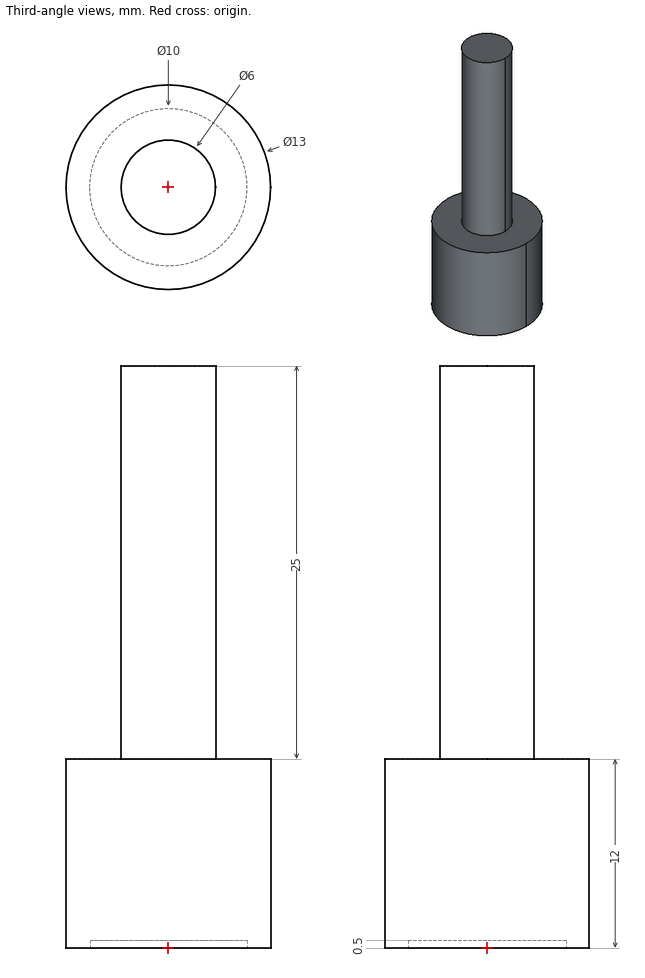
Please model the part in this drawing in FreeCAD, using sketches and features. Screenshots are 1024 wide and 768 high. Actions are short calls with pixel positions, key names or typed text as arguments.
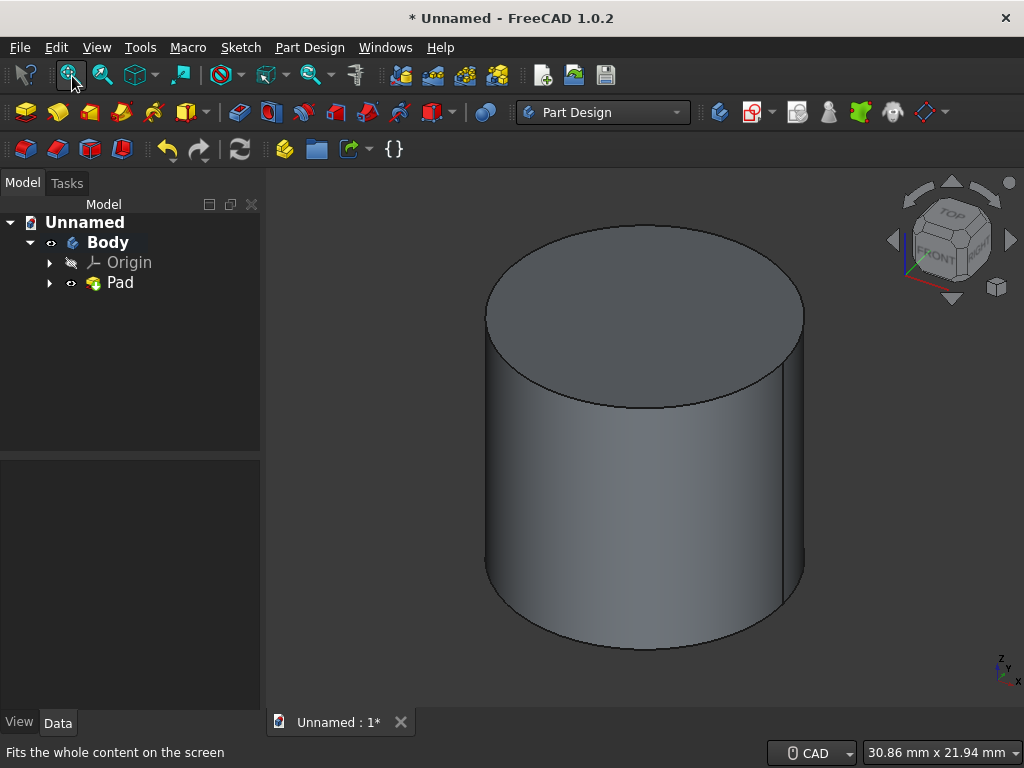
click(645, 316)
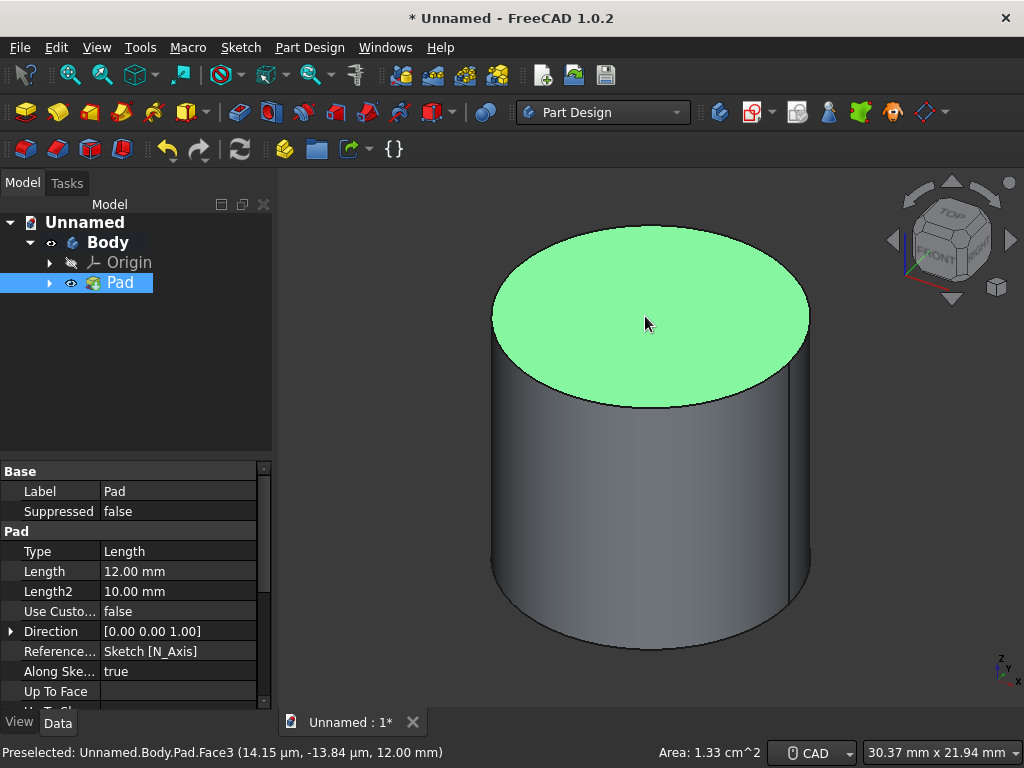
click(752, 112)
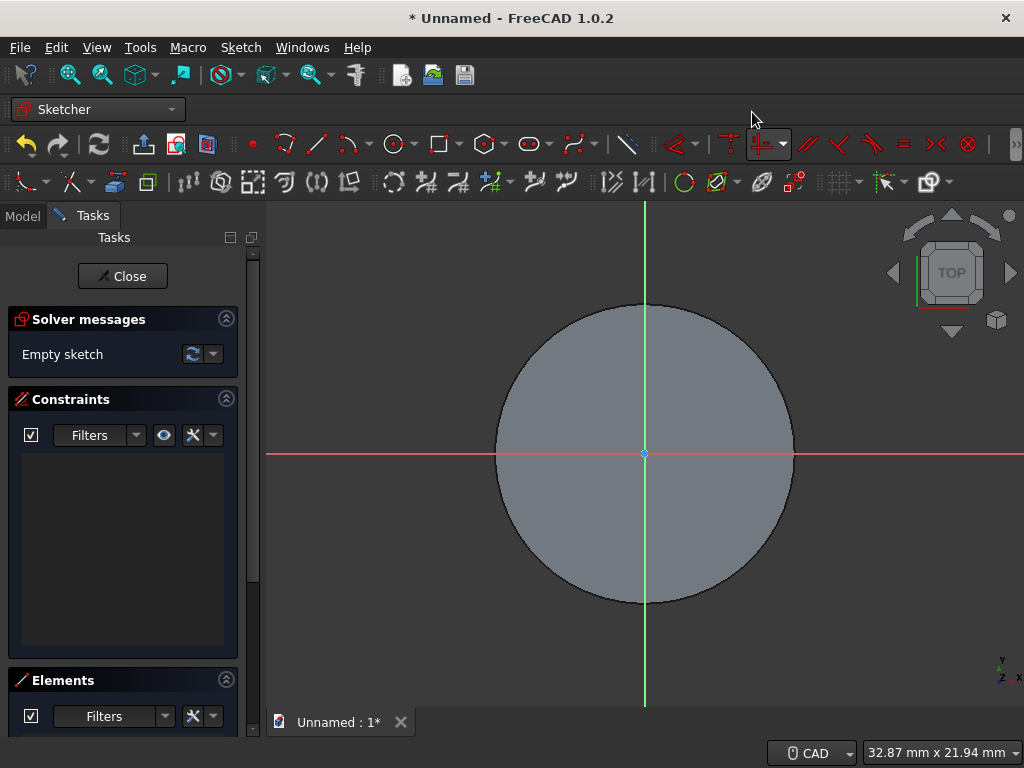
scroll(701, 454, up, 4)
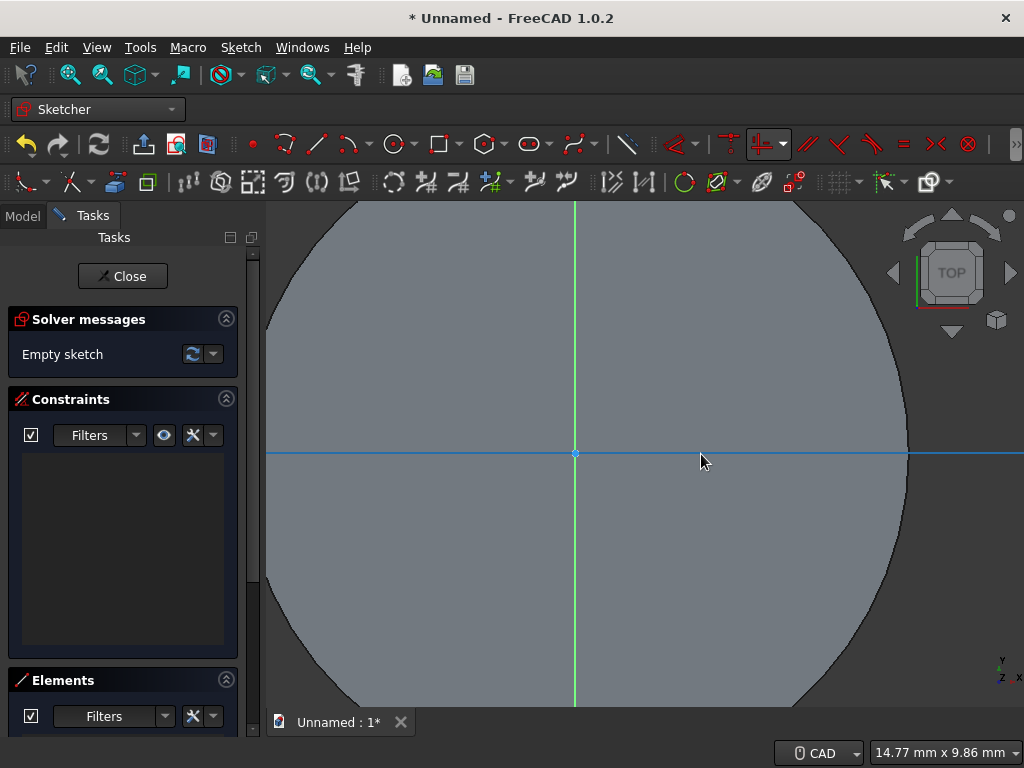
click(394, 144)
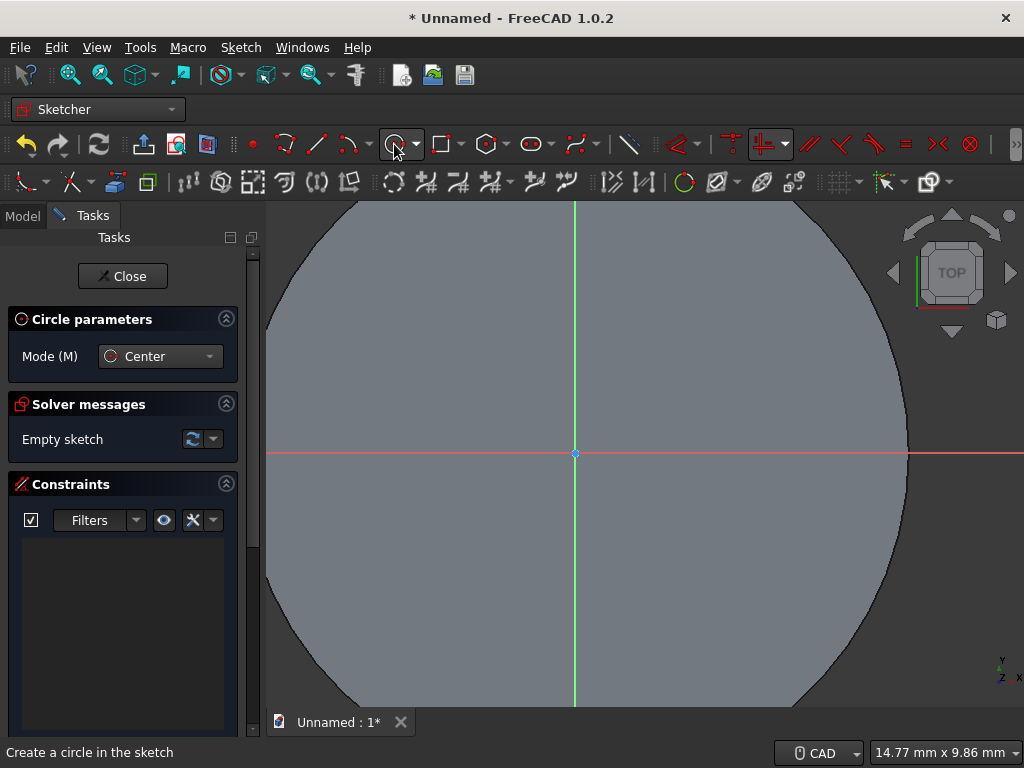
click(575, 453)
move(684, 345)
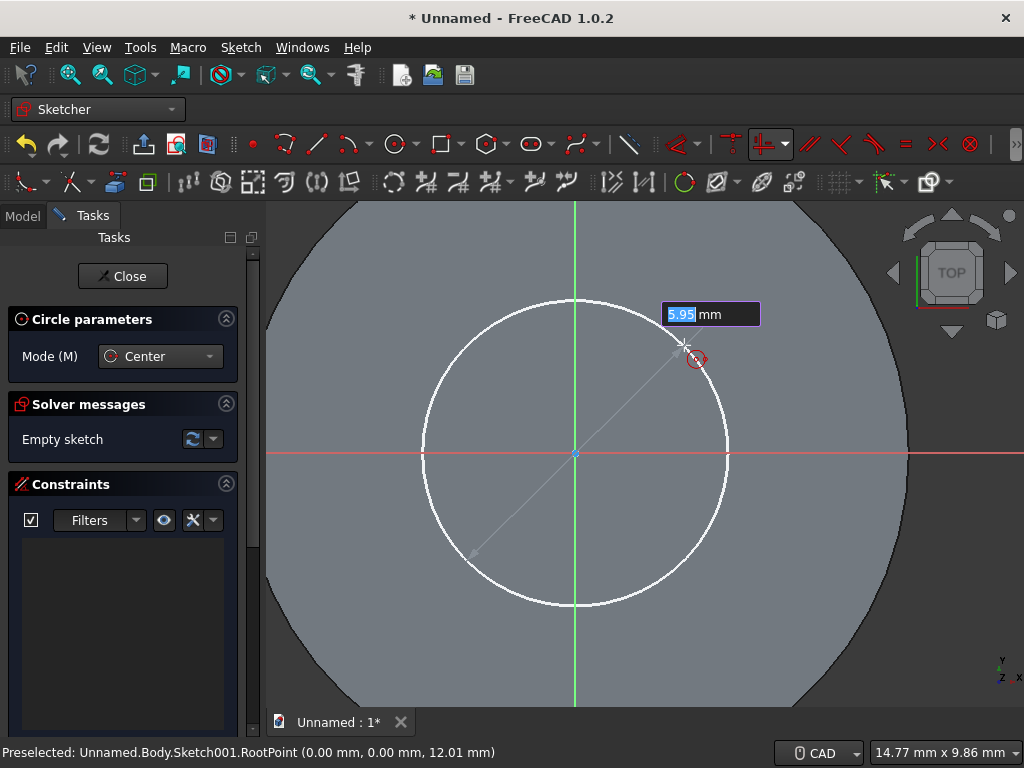
text(6)
key(Return)
key(Escape)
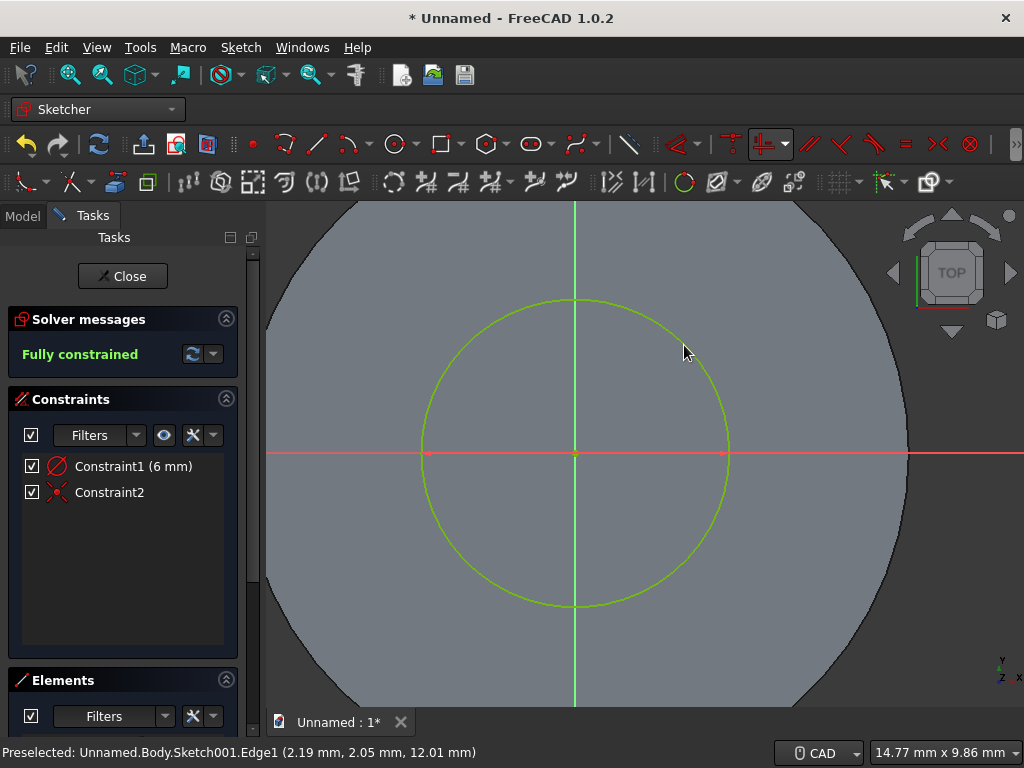
click(123, 276)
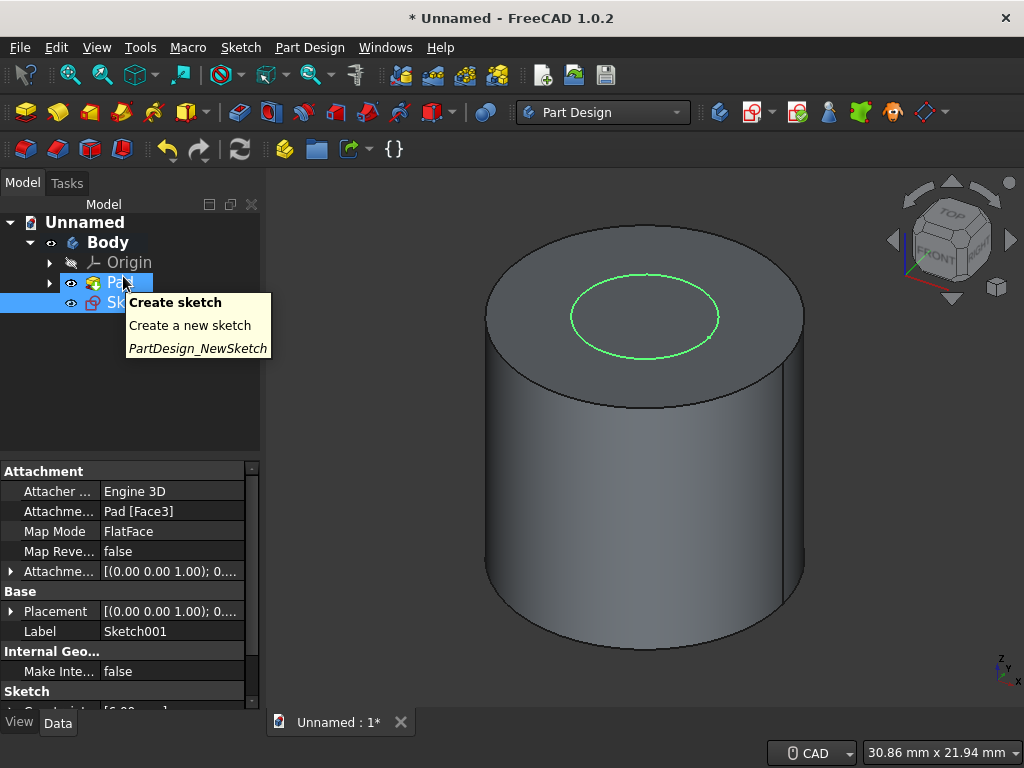
click(26, 112)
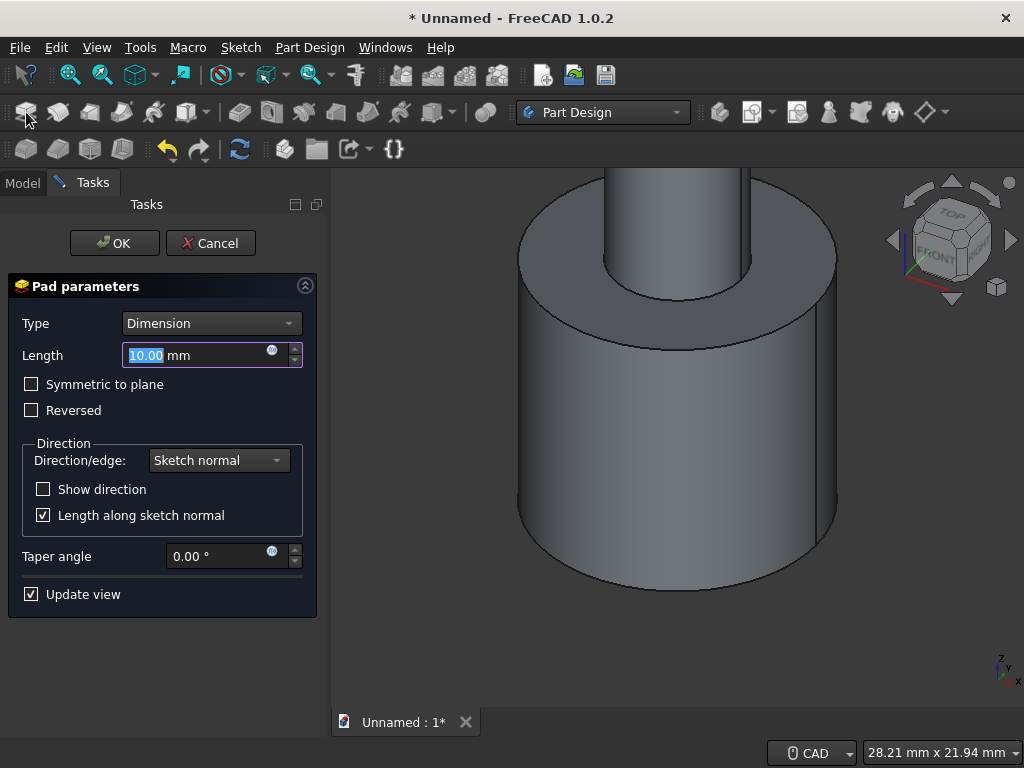
text(25)
key(Tab)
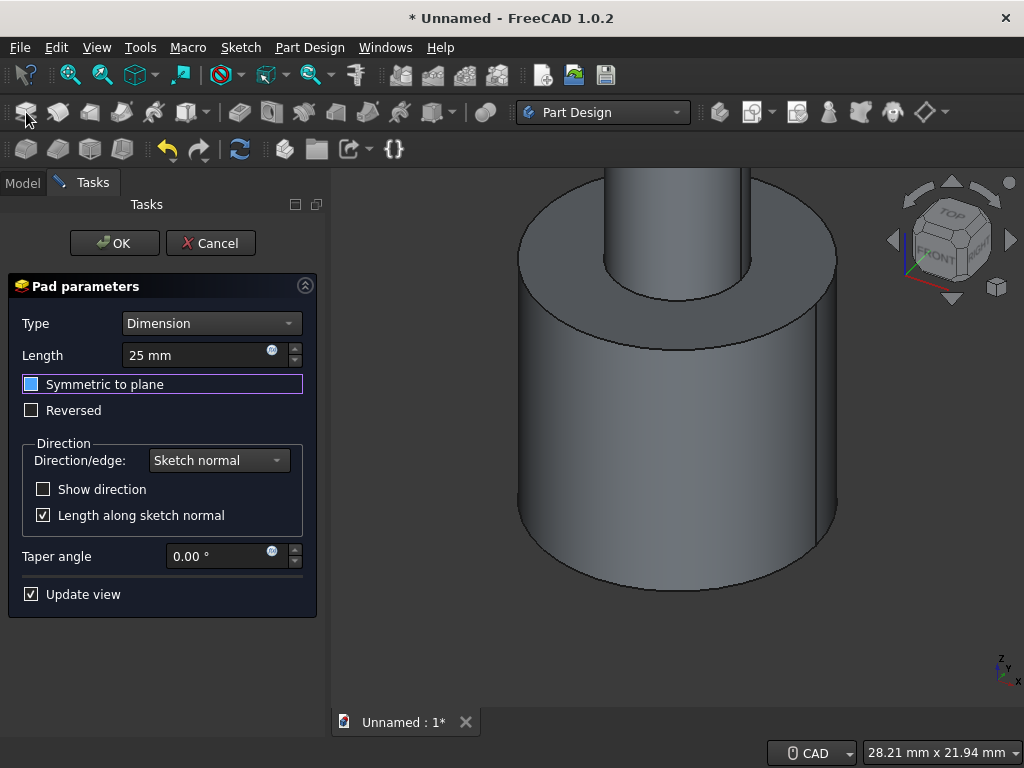
click(115, 243)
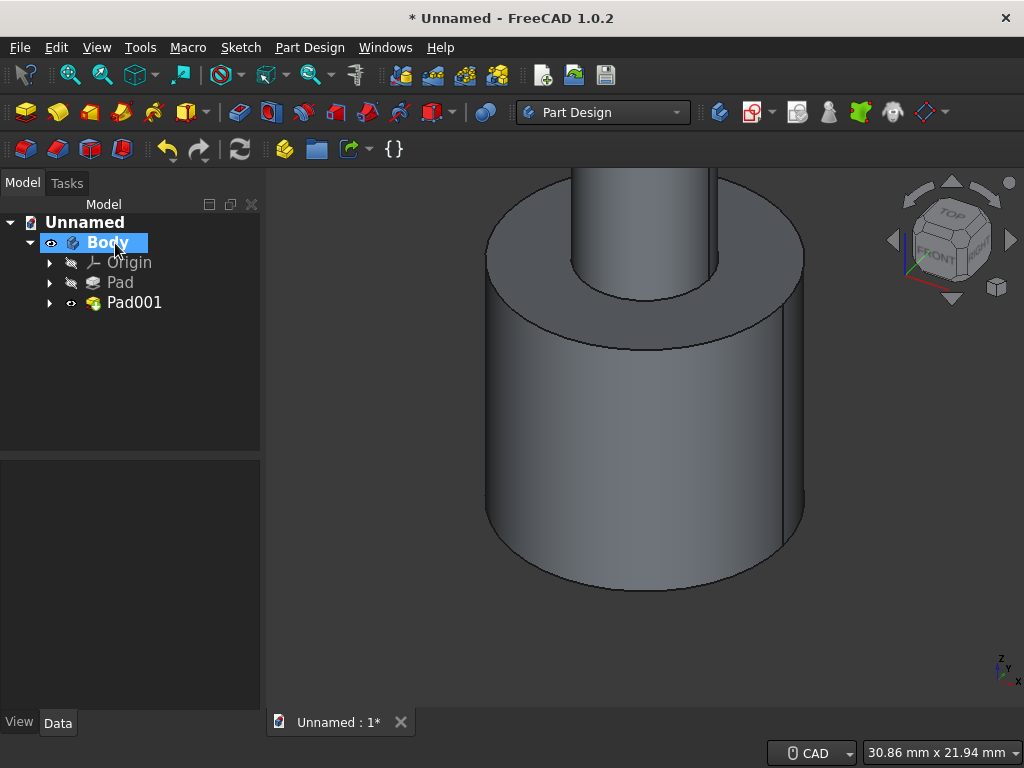
click(72, 76)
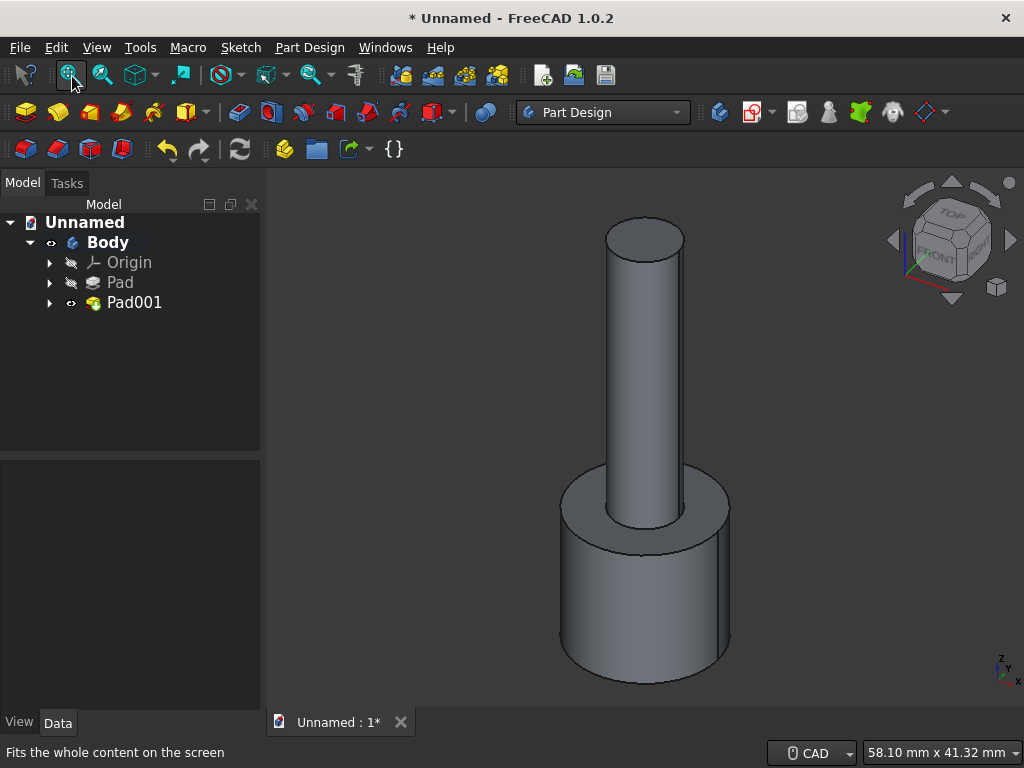
key(5)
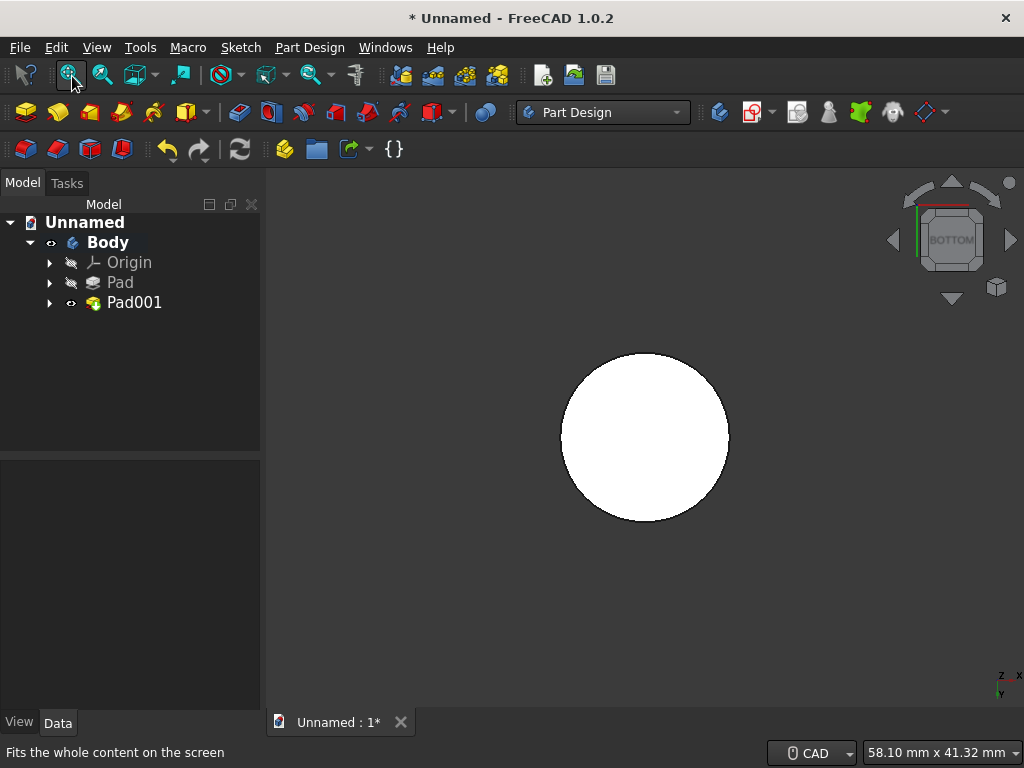
click(72, 76)